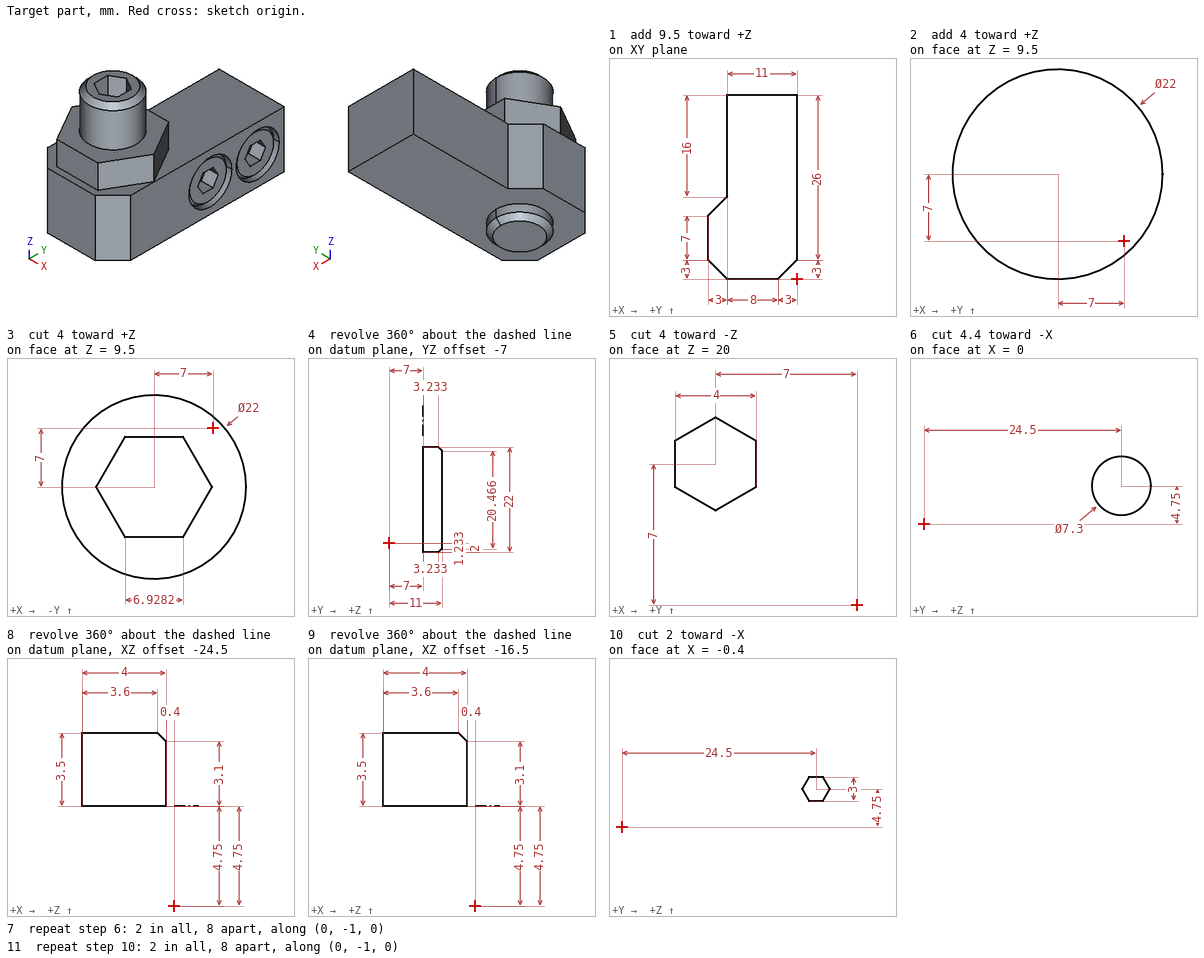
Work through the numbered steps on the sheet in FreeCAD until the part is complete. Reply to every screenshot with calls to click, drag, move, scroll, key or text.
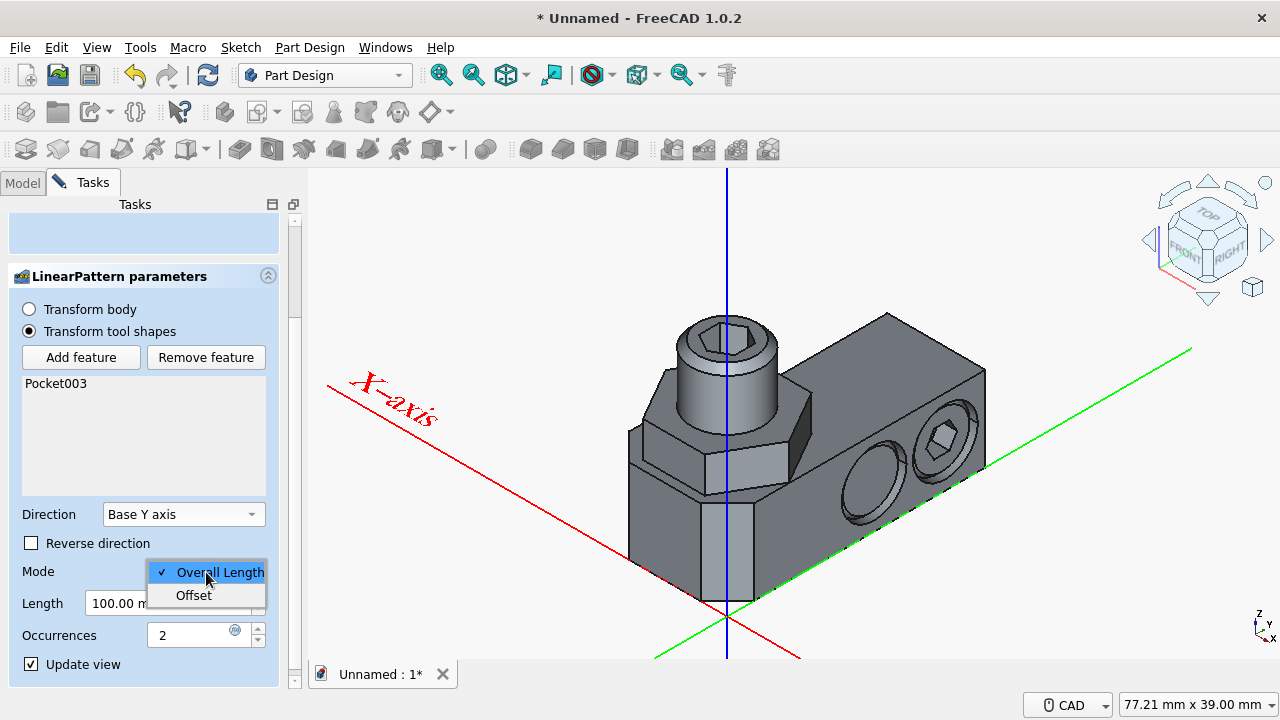
click(206, 596)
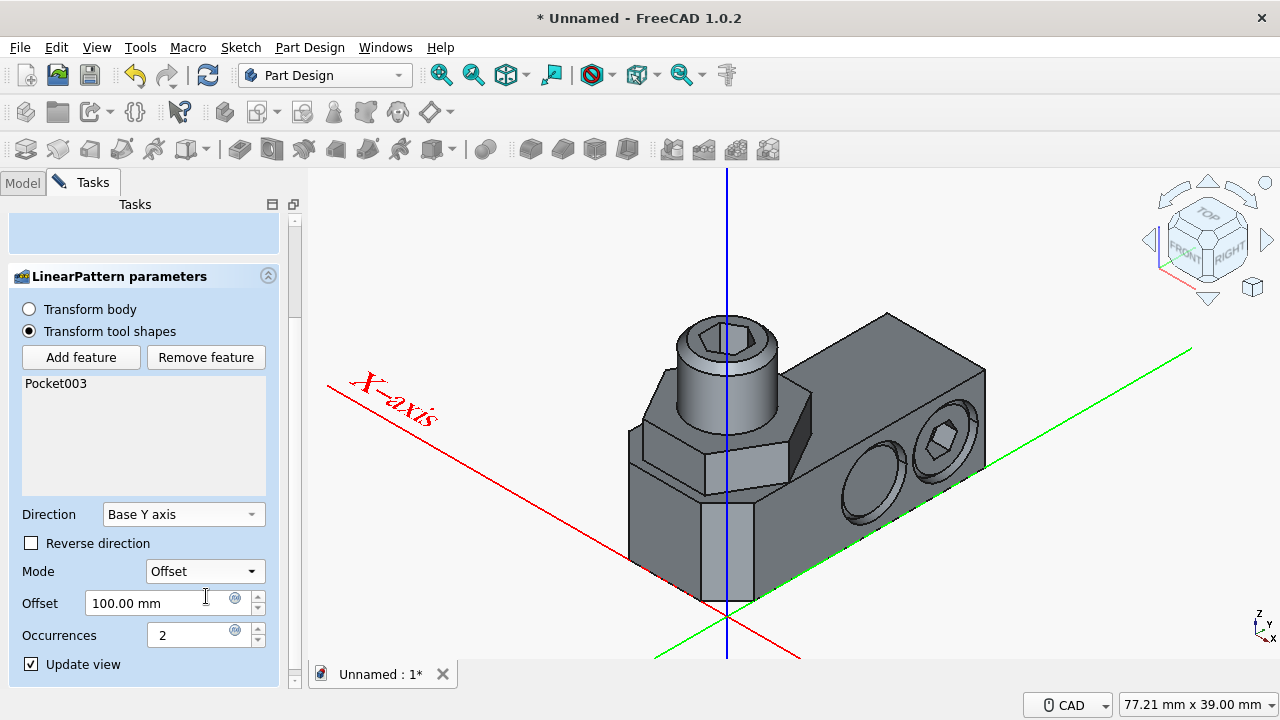
triple_click(168, 603)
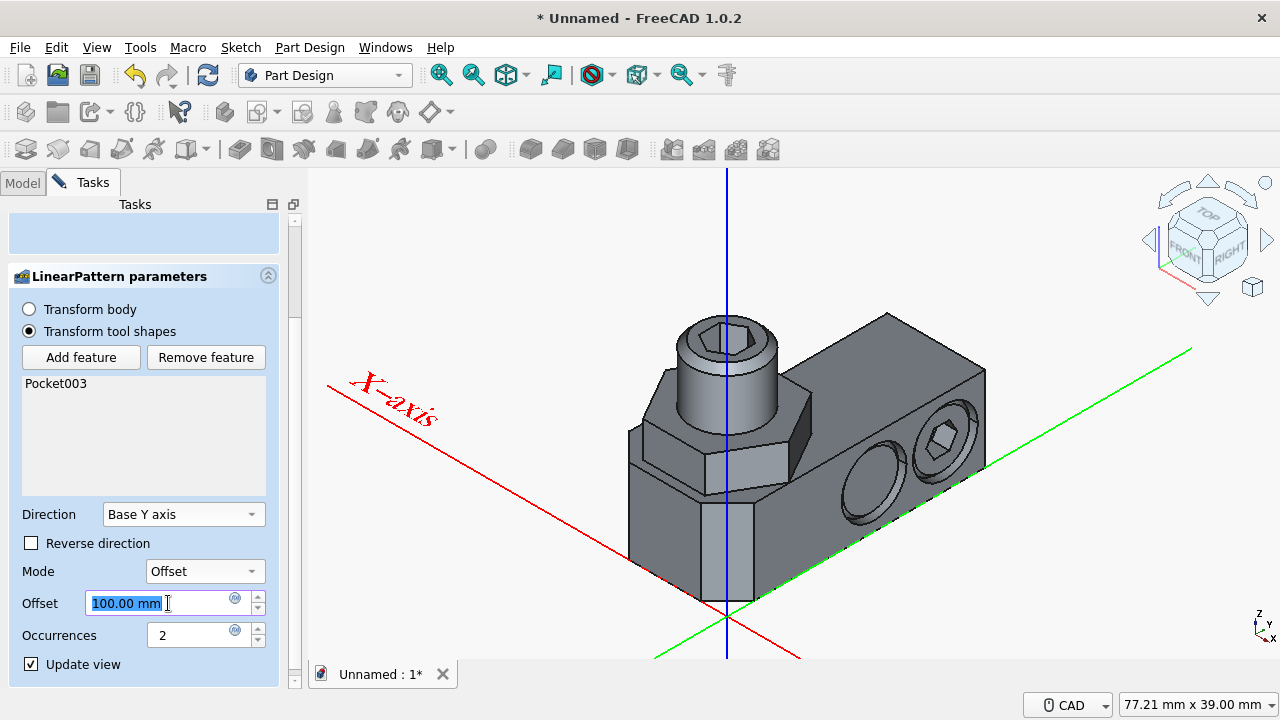
text(8)
key(Tab)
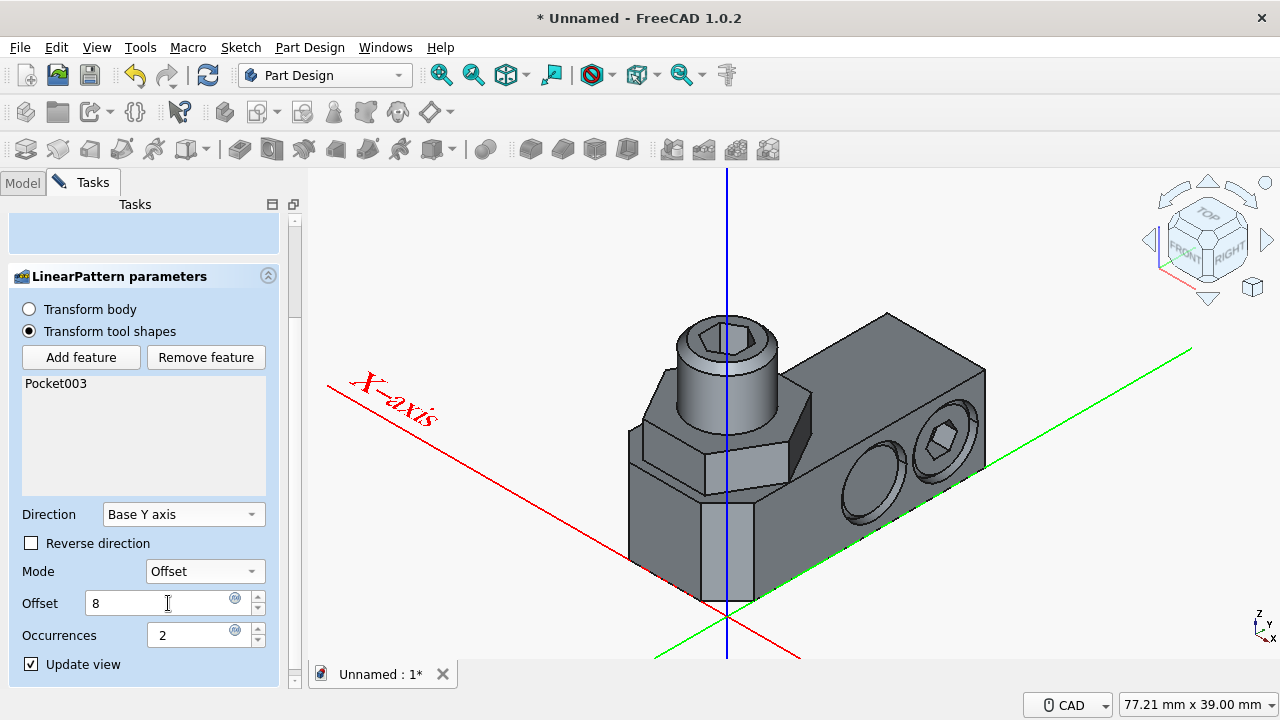
triple_click(198, 635)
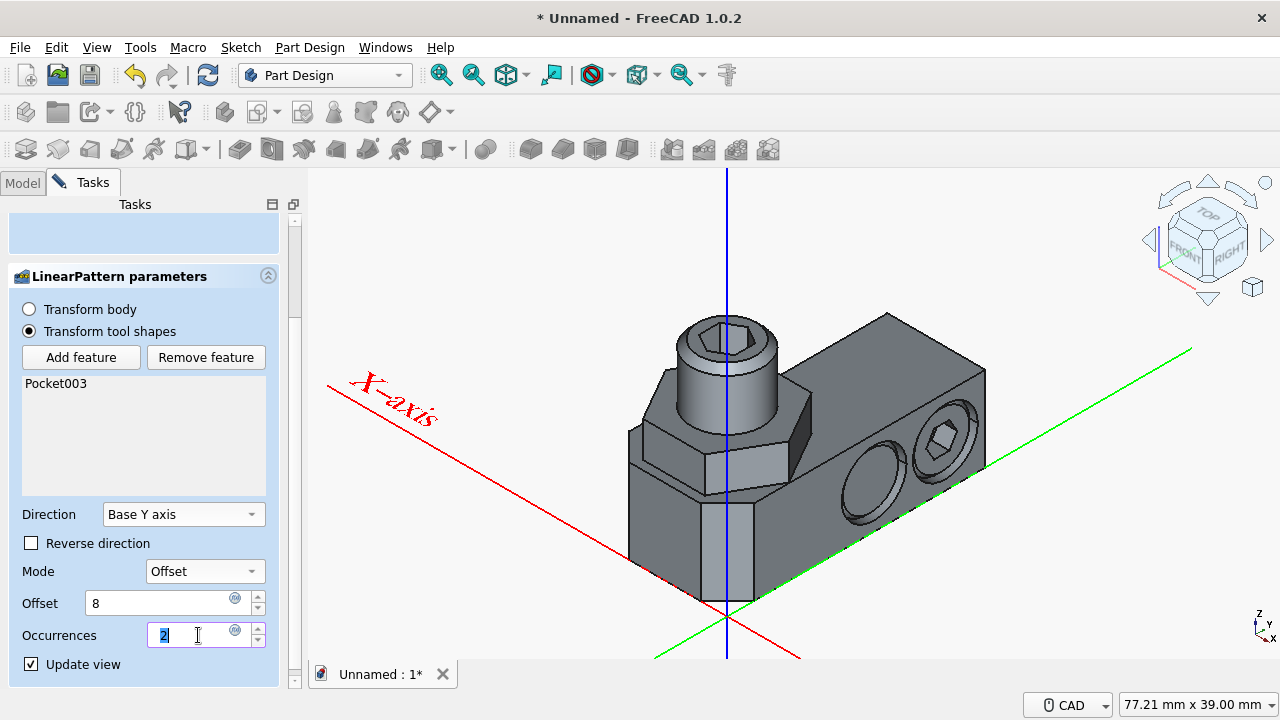
text(2)
key(Tab)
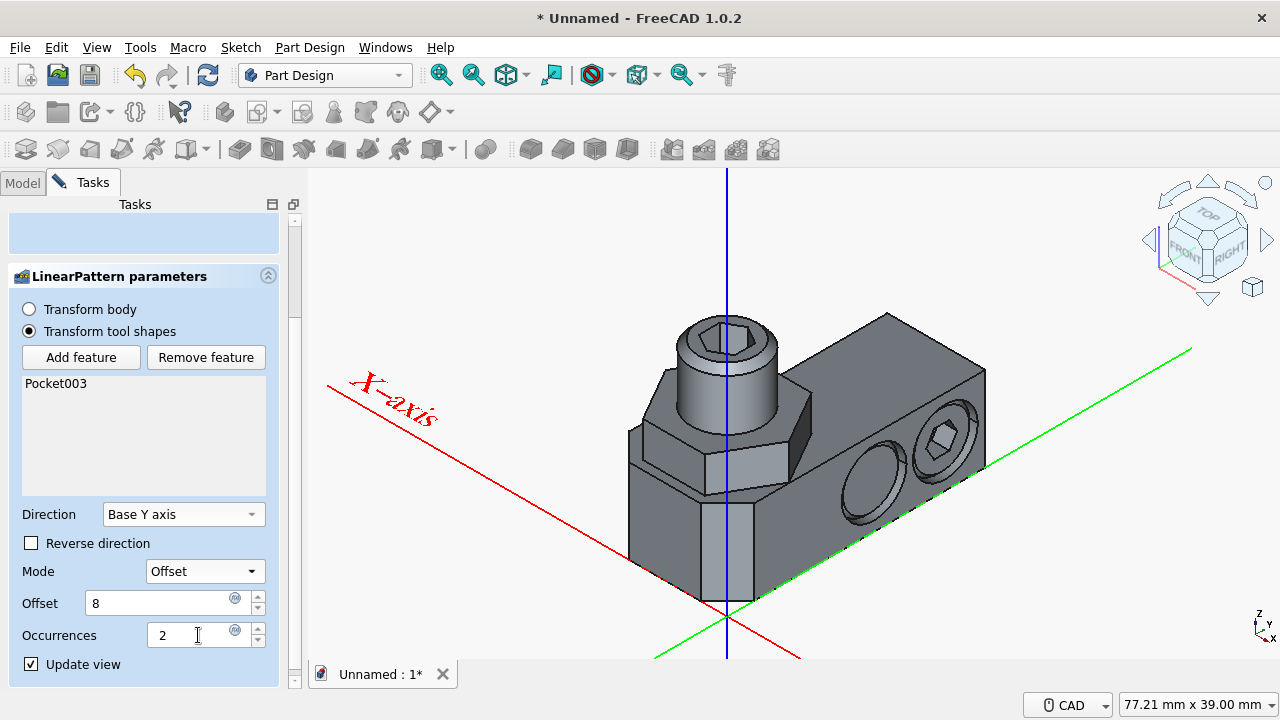
click(30, 543)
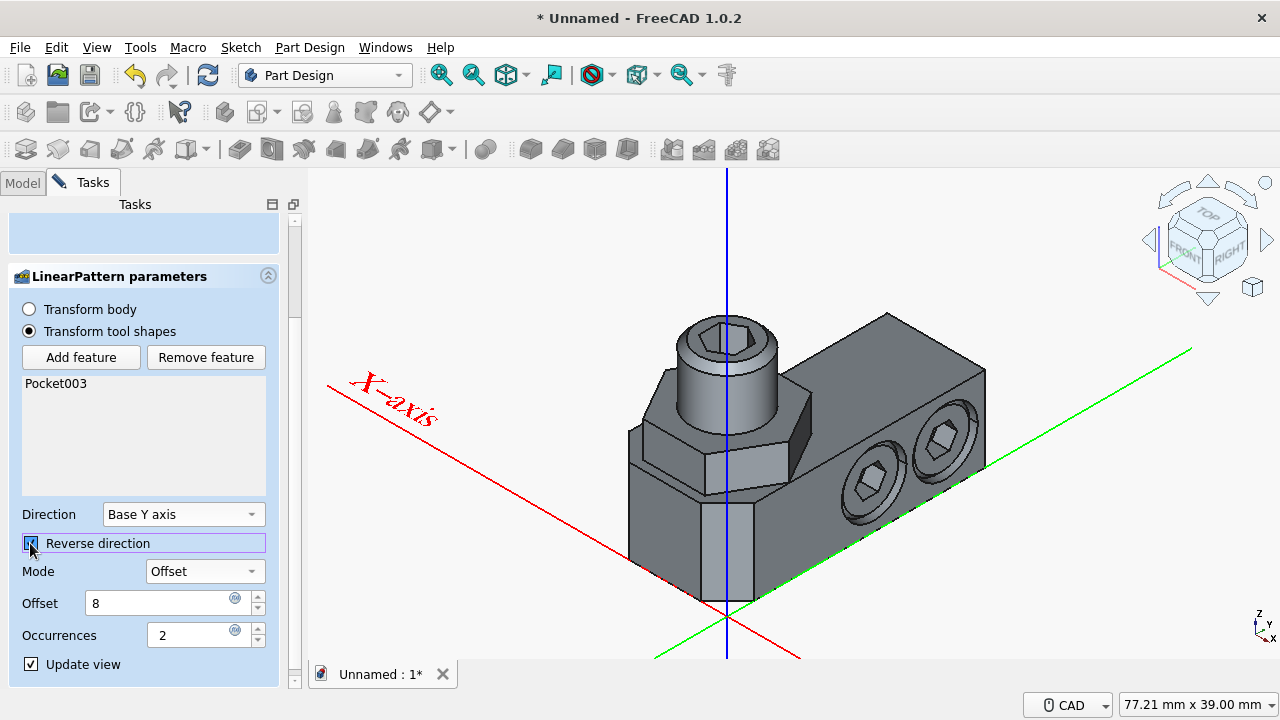
scroll(295, 451, up, 3)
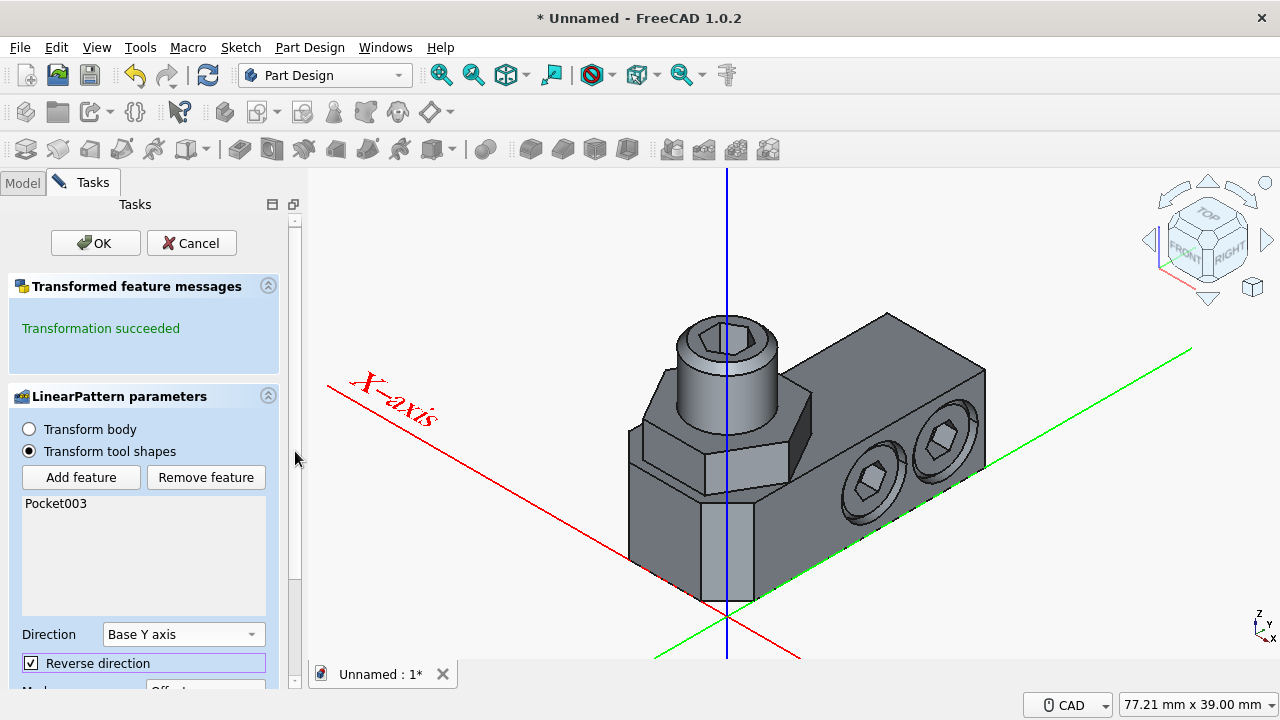
click(96, 243)